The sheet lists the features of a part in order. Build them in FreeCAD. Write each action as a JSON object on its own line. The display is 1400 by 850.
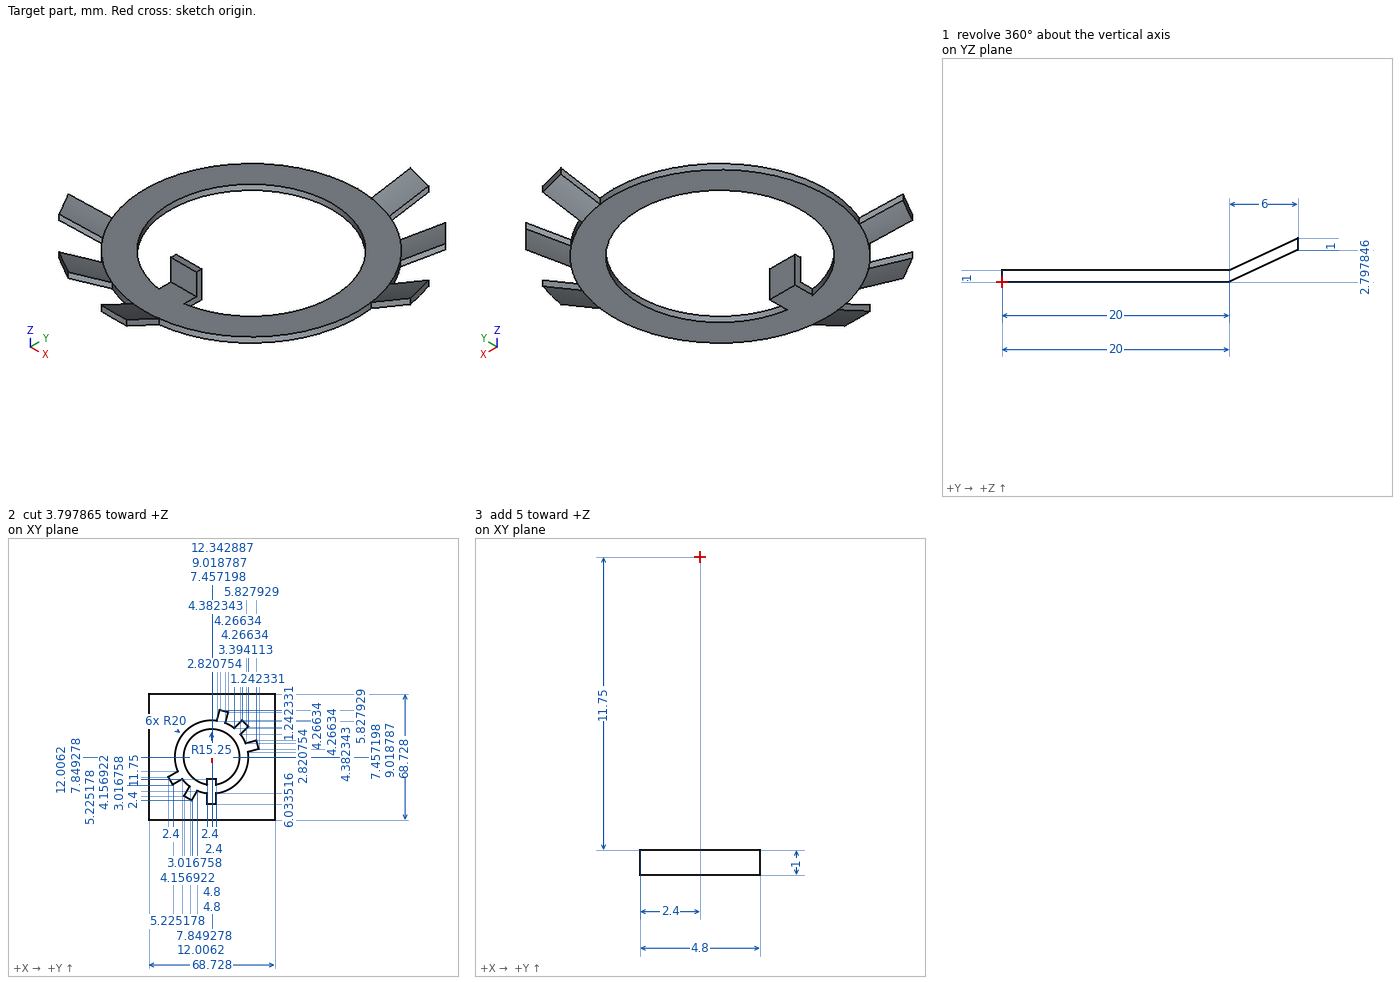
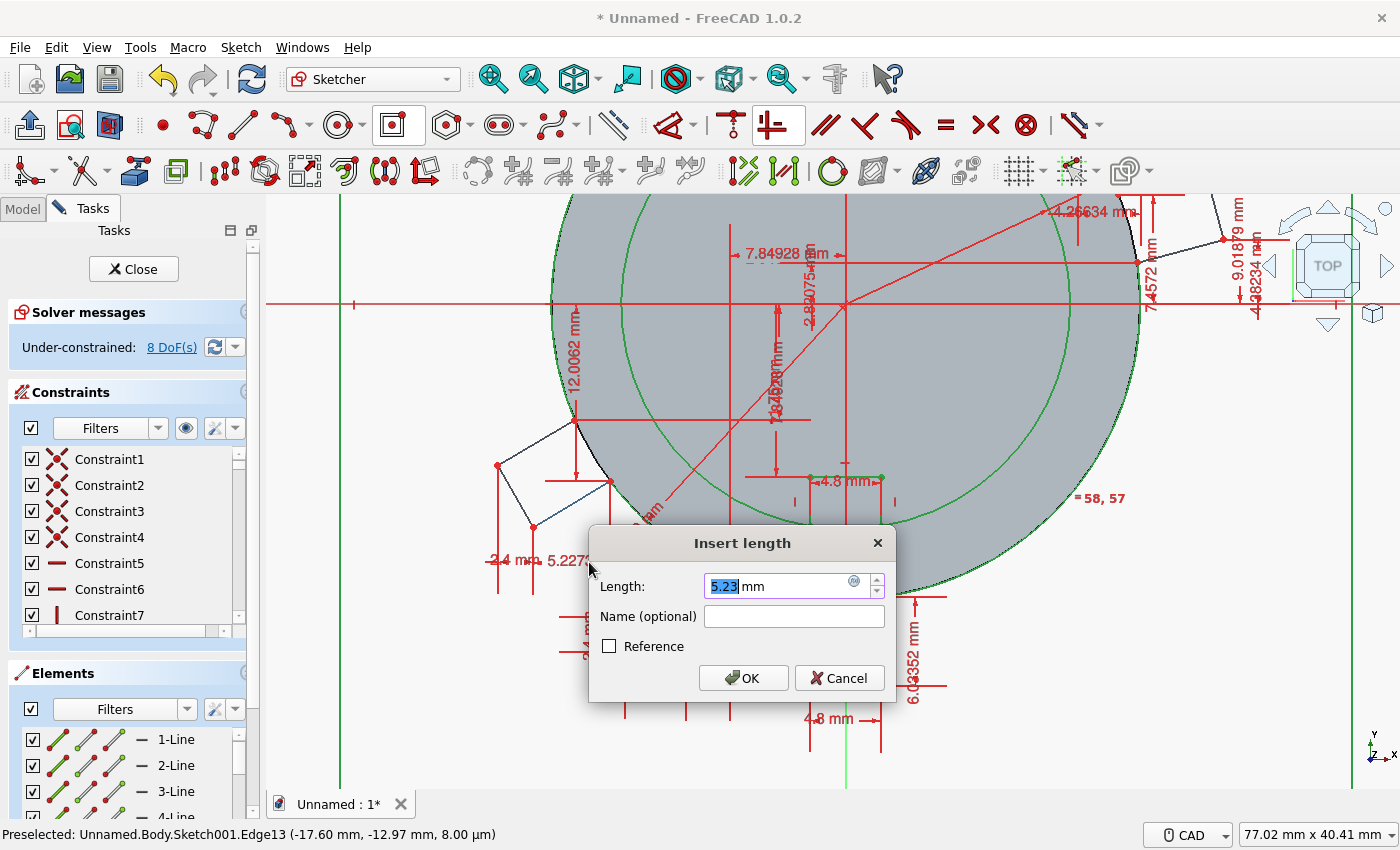
{"action": "type", "text": "5.225178"}
{"action": "key", "text": "Return"}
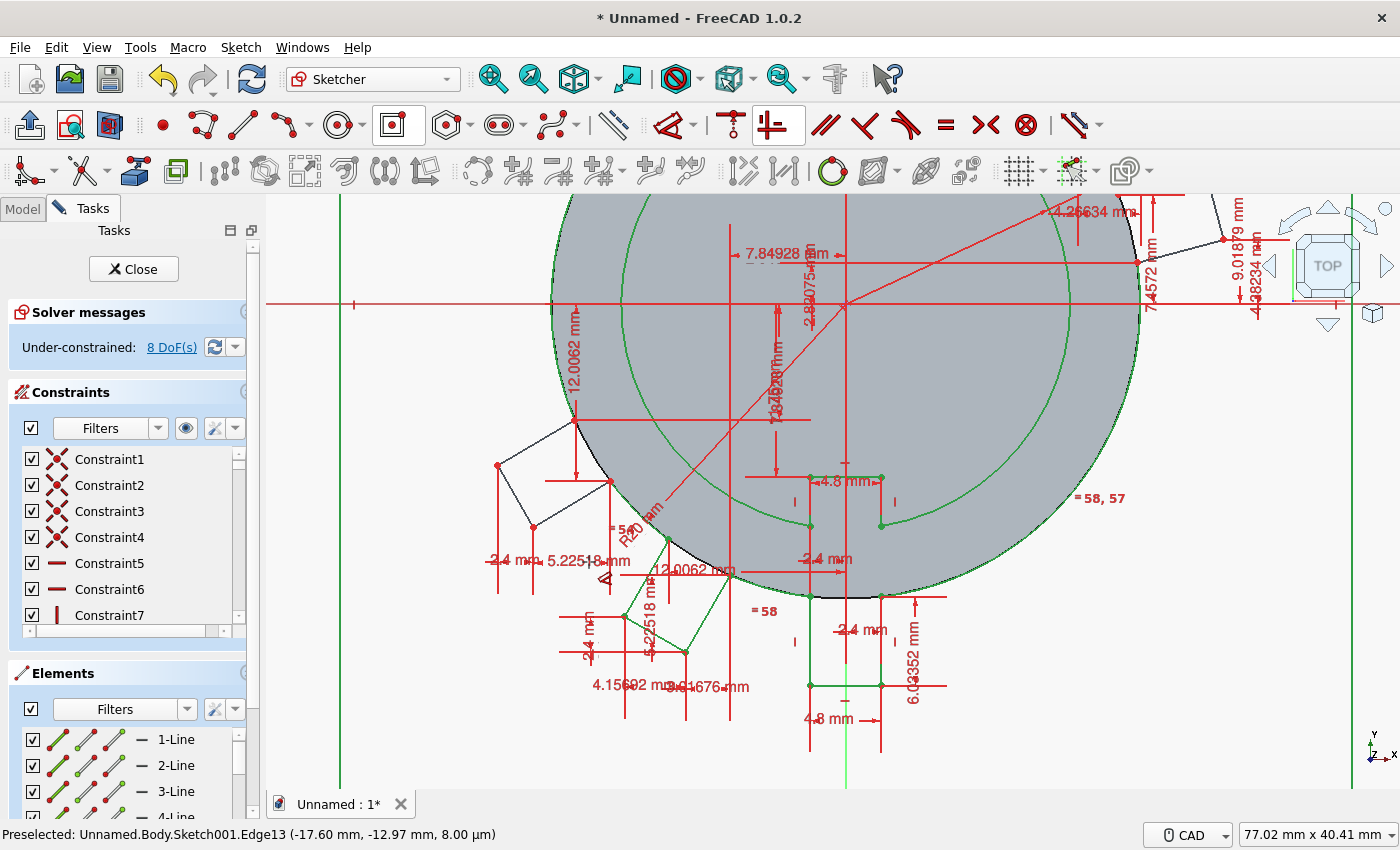
{"action": "left_click", "coordinate": [587, 495]}
{"action": "left_click", "coordinate": [499, 504]}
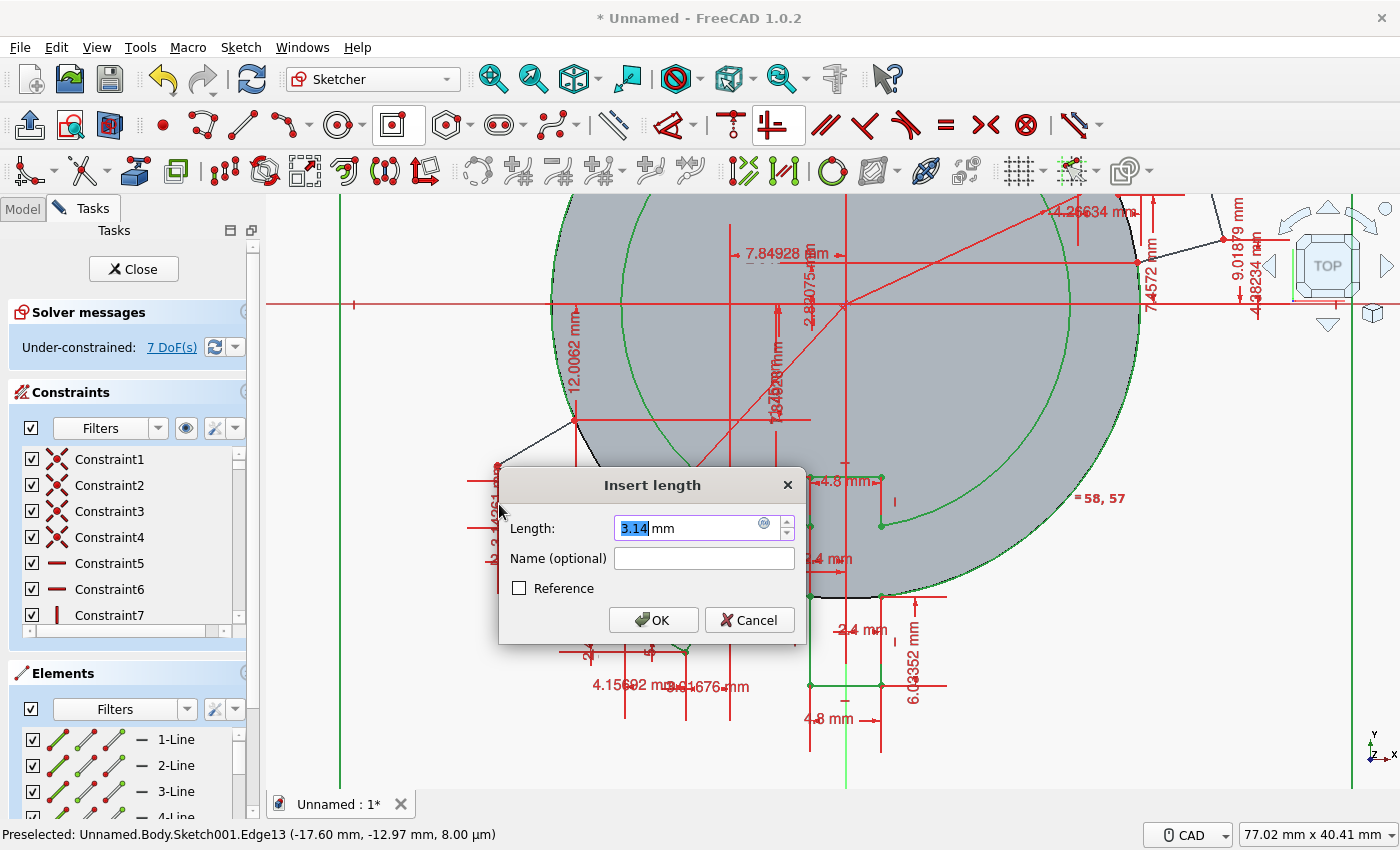
{"action": "type", "text": "3.016758"}
{"action": "key", "text": "Return"}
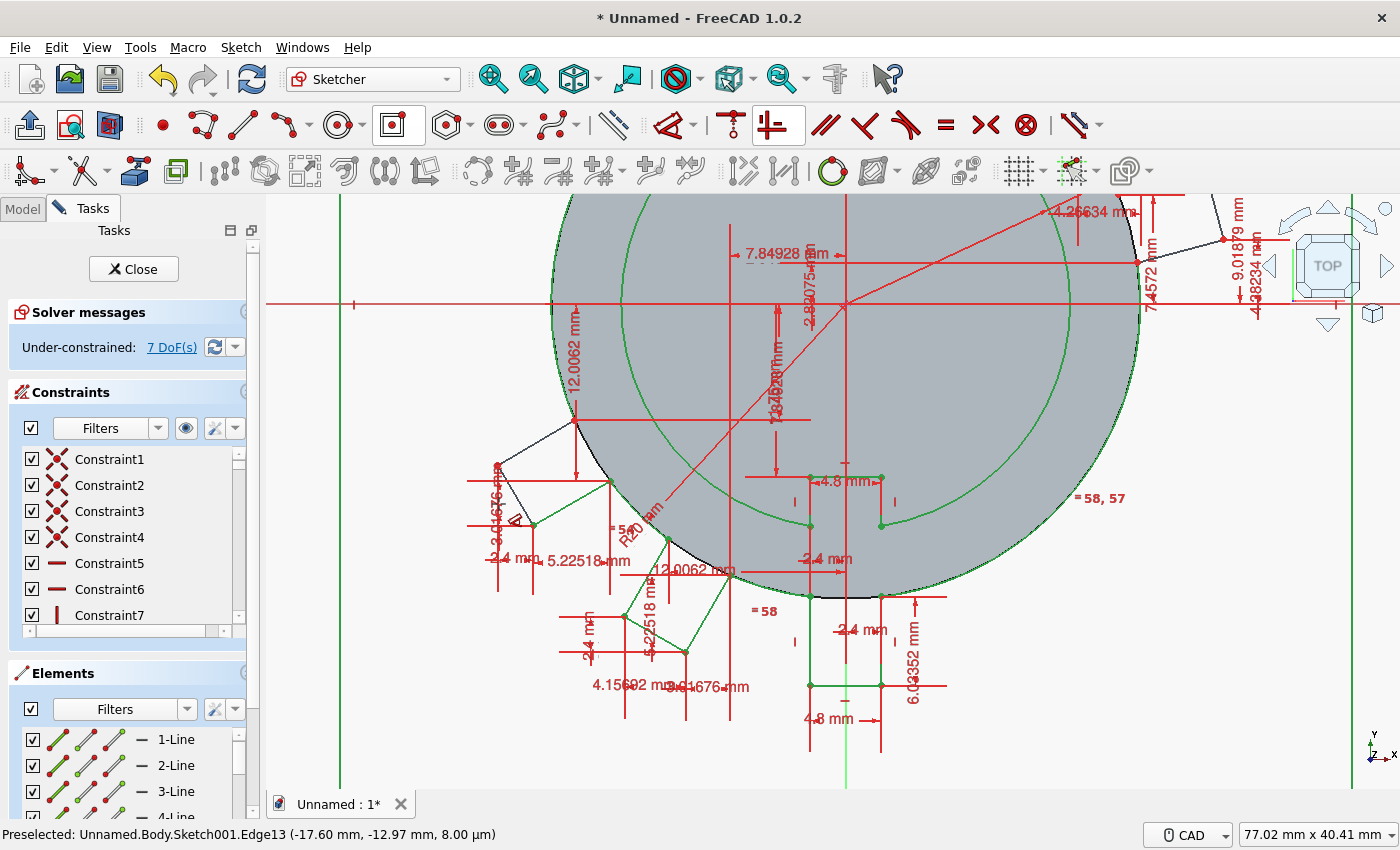
{"action": "left_click", "coordinate": [523, 508]}
{"action": "left_click", "coordinate": [464, 482]}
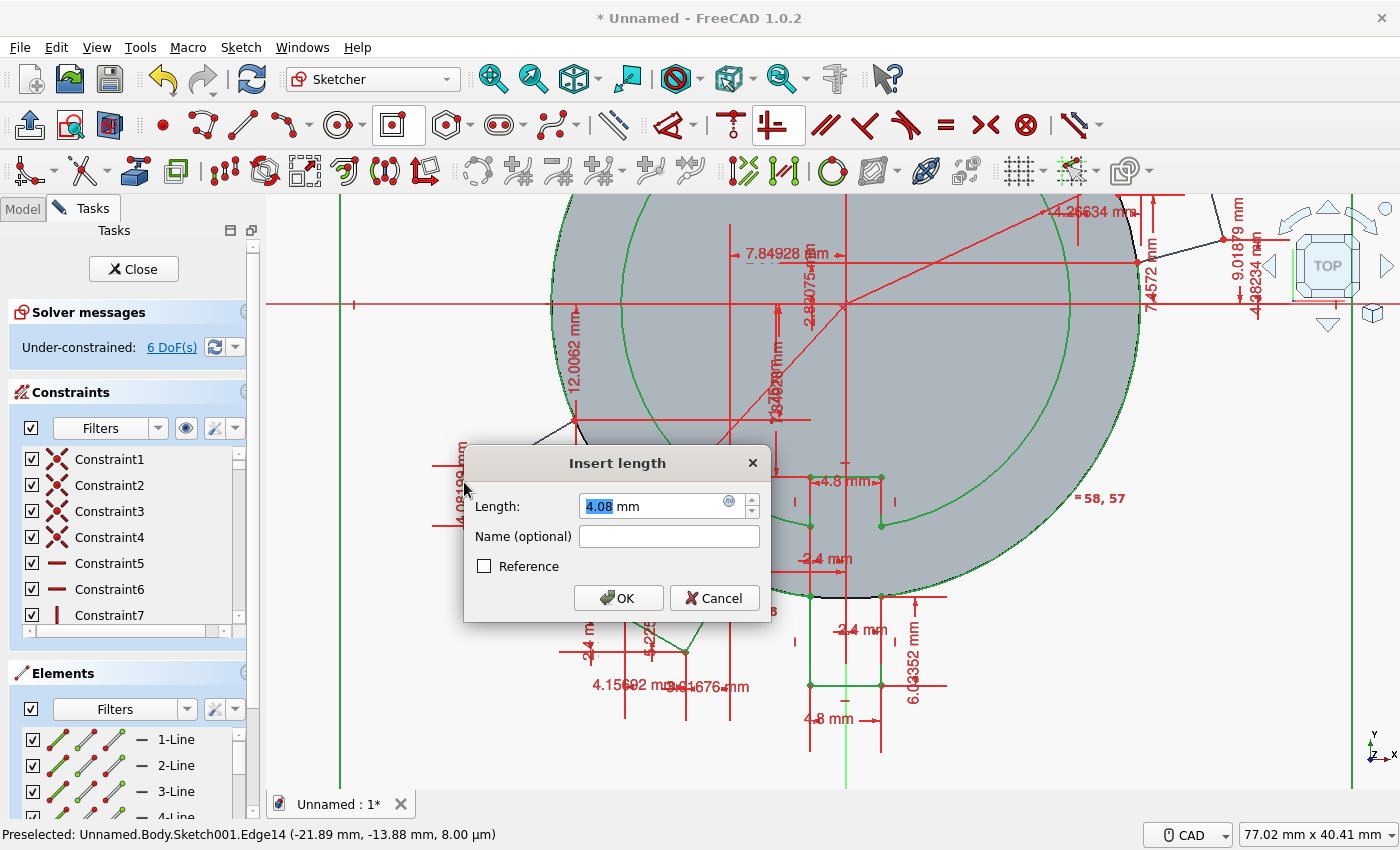
{"action": "type", "text": "4.156922"}
{"action": "key", "text": "Return"}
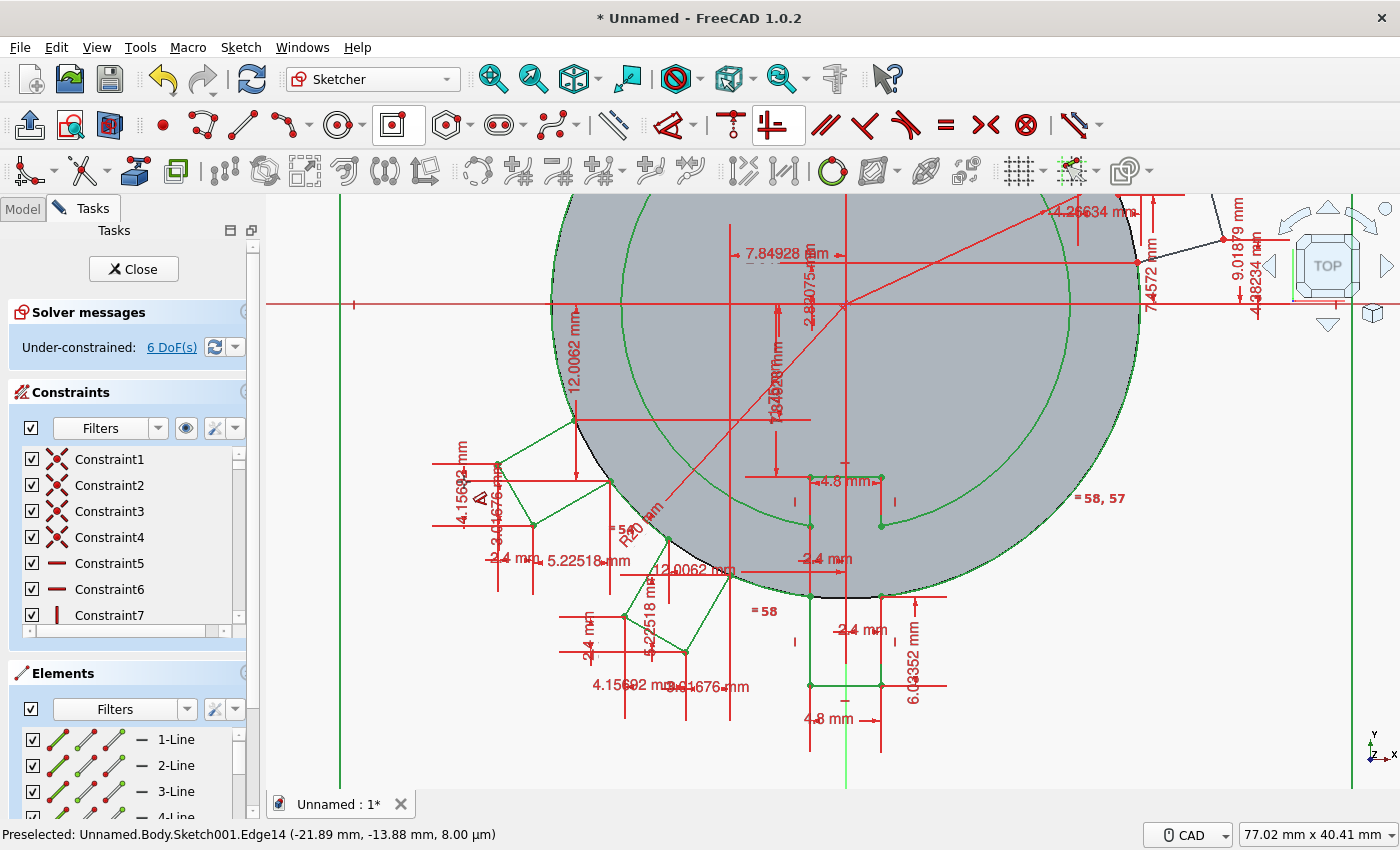
{"action": "scroll", "coordinate": [717, 600], "scroll_direction": "down", "scroll_amount": 5}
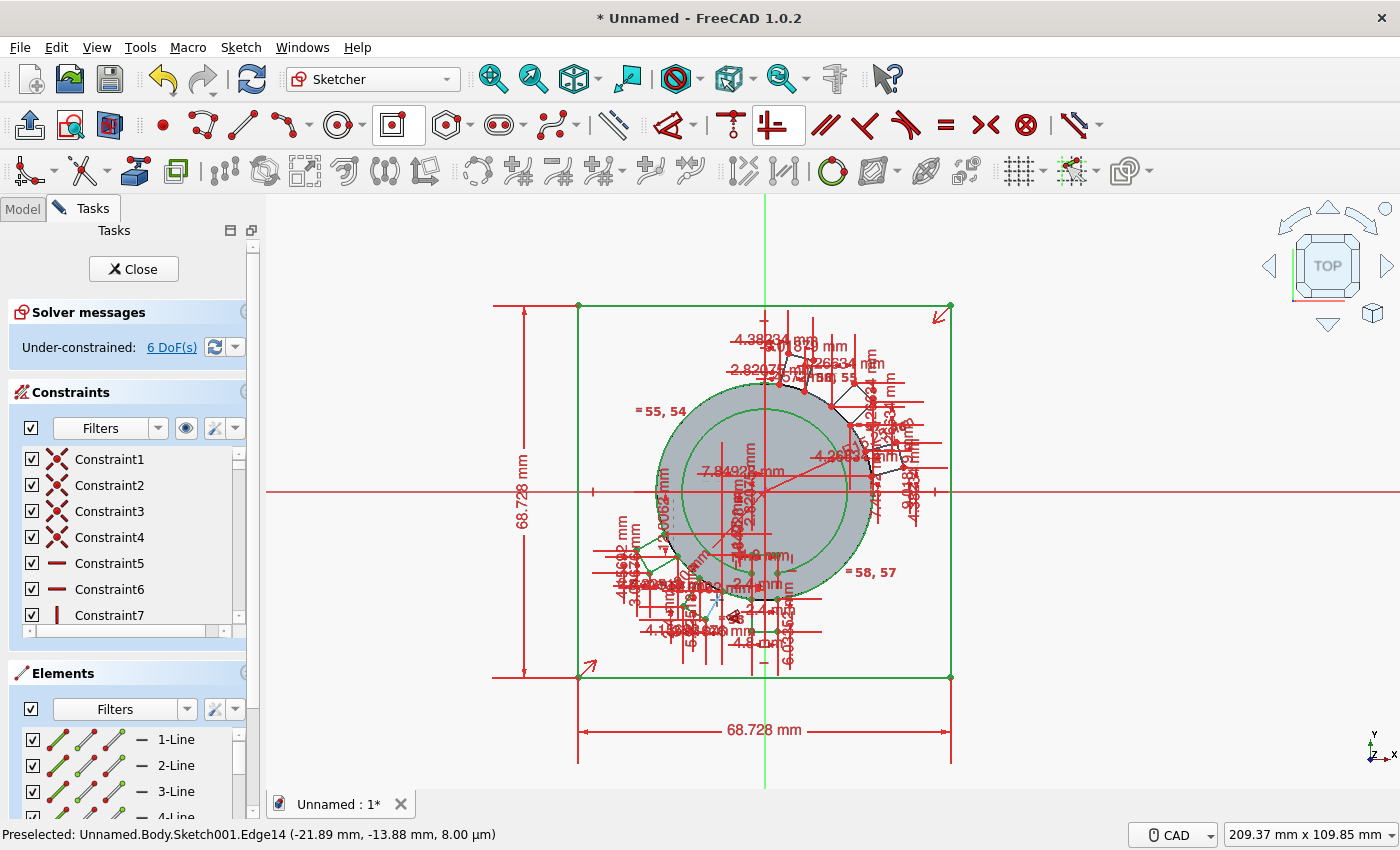
{"action": "scroll", "coordinate": [782, 375], "scroll_direction": "up", "scroll_amount": 2}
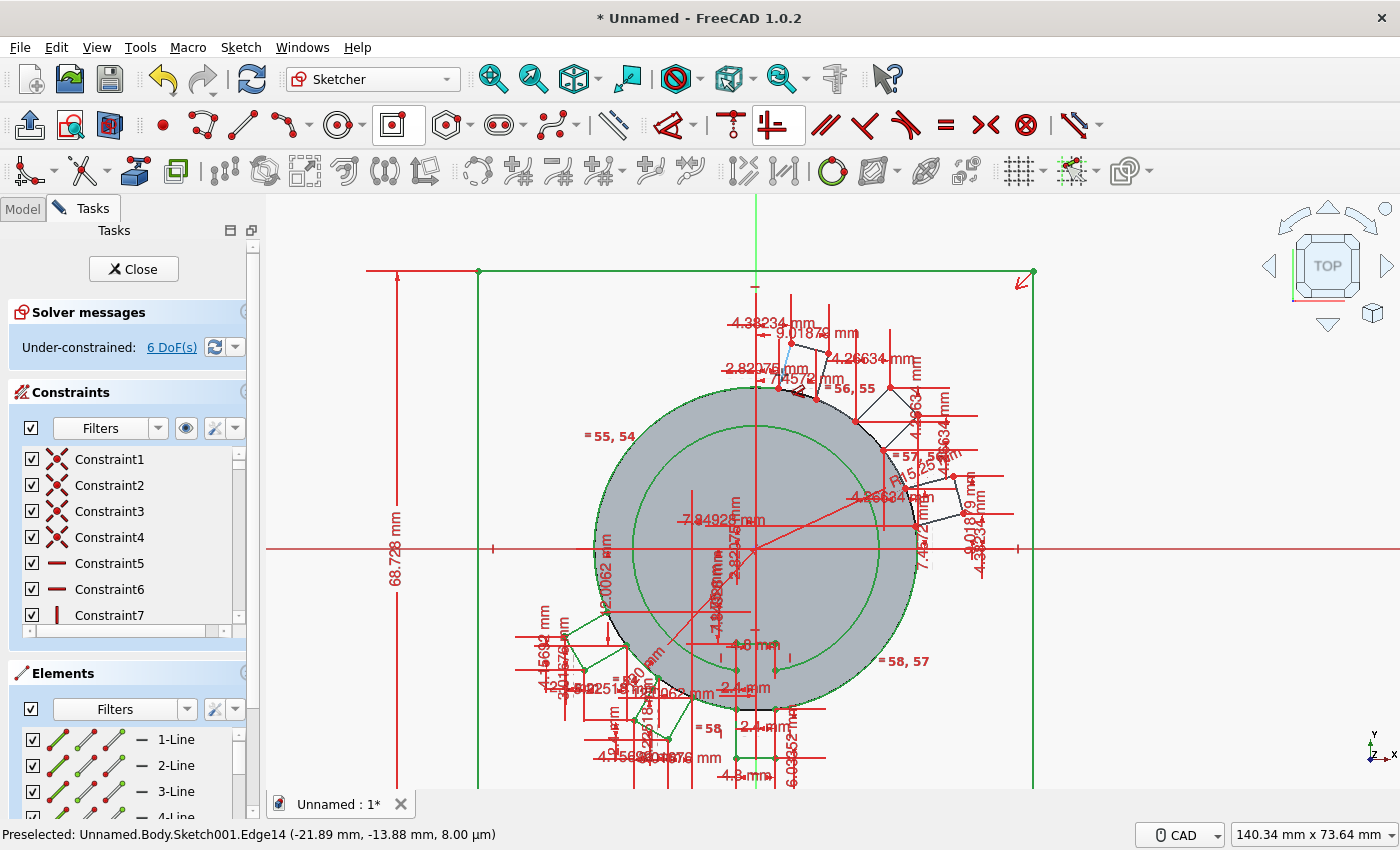
{"action": "left_click", "coordinate": [782, 375]}
{"action": "left_click", "coordinate": [721, 350]}